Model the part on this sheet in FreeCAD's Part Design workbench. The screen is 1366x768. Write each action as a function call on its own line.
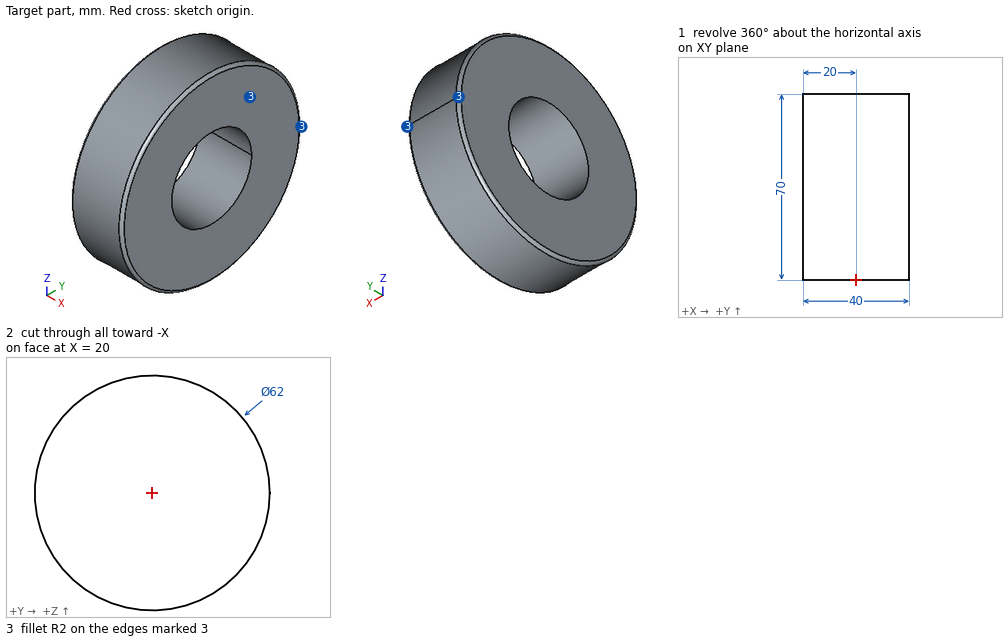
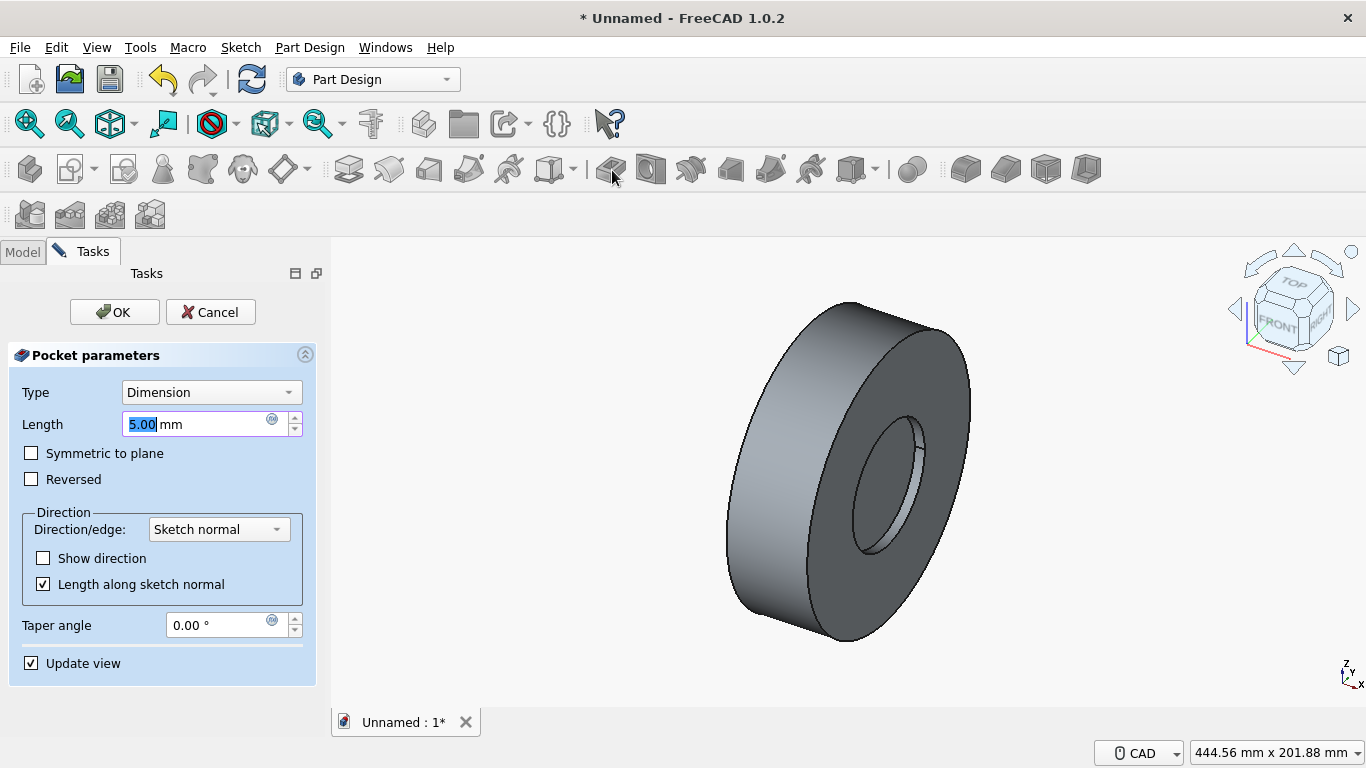
click(212, 392)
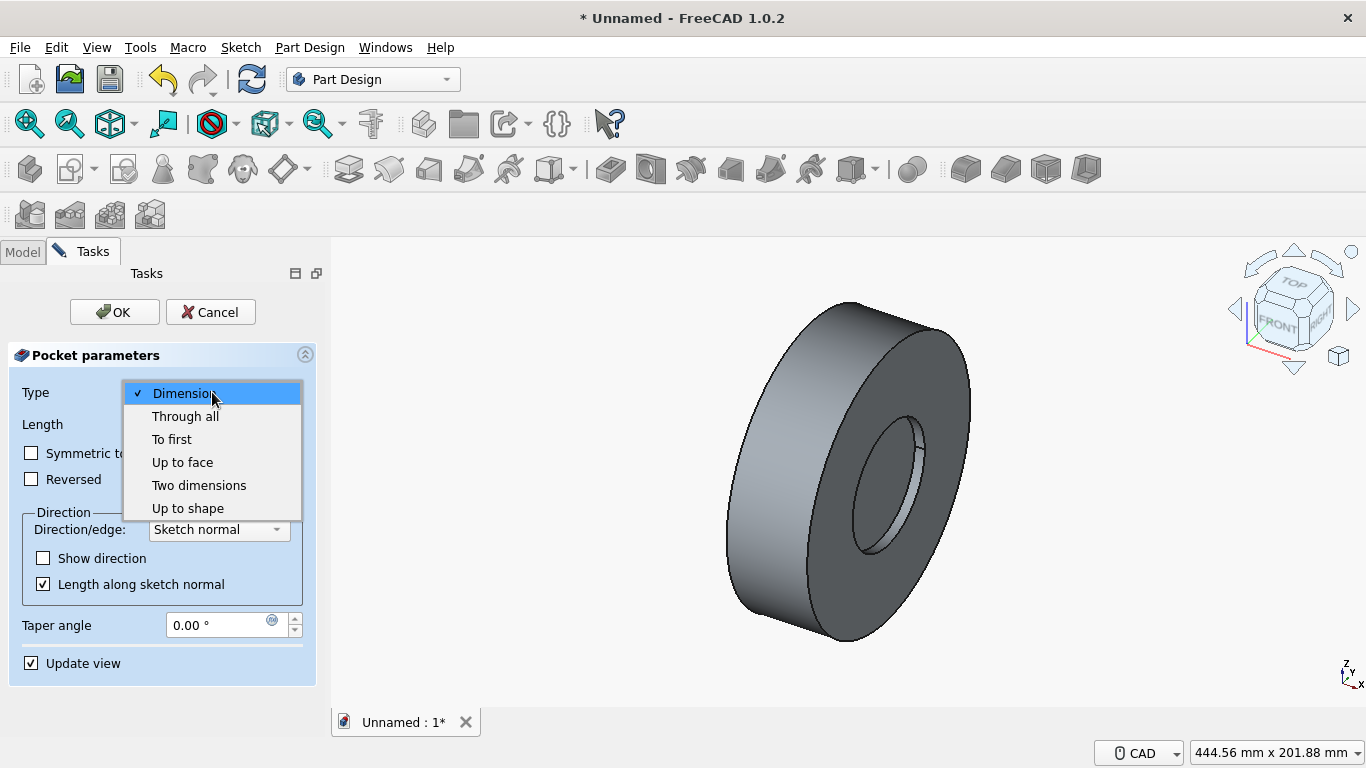
click(212, 416)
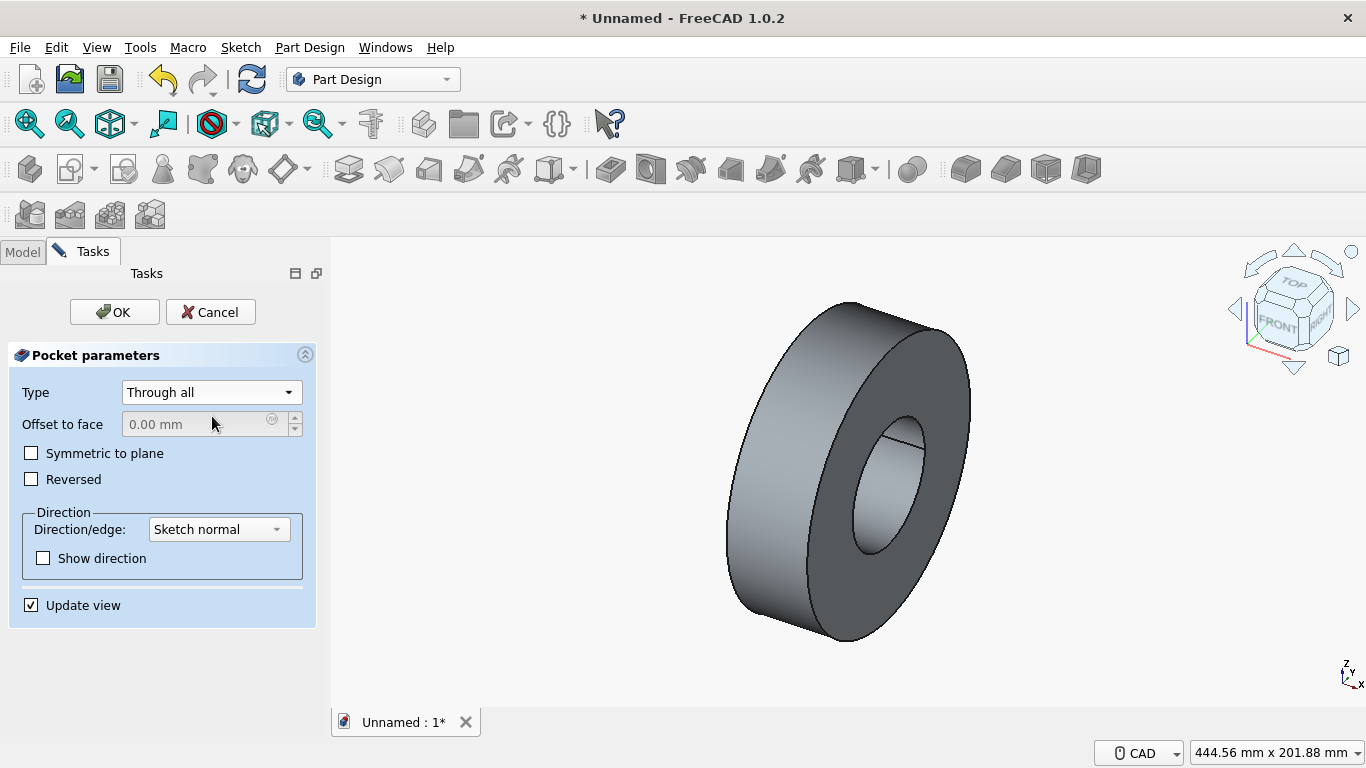
click(115, 312)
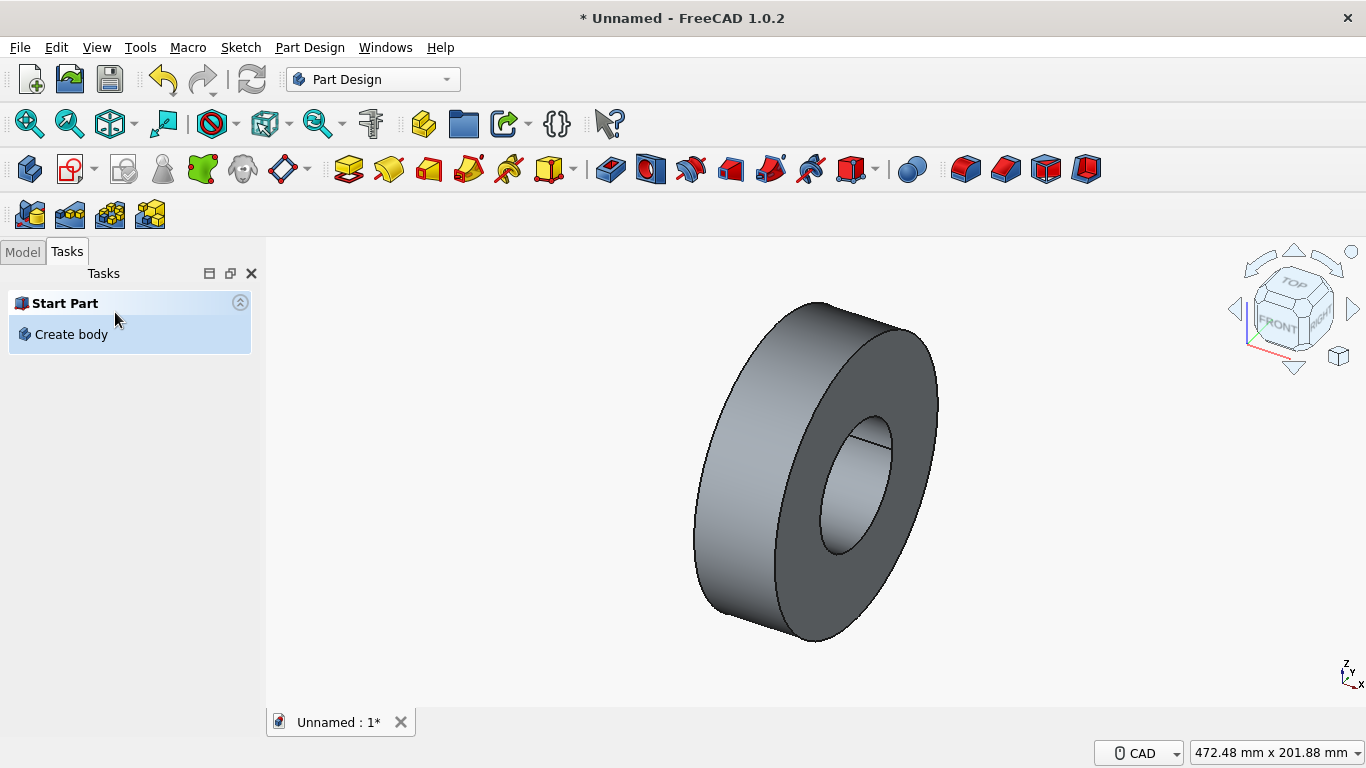
click(775, 565)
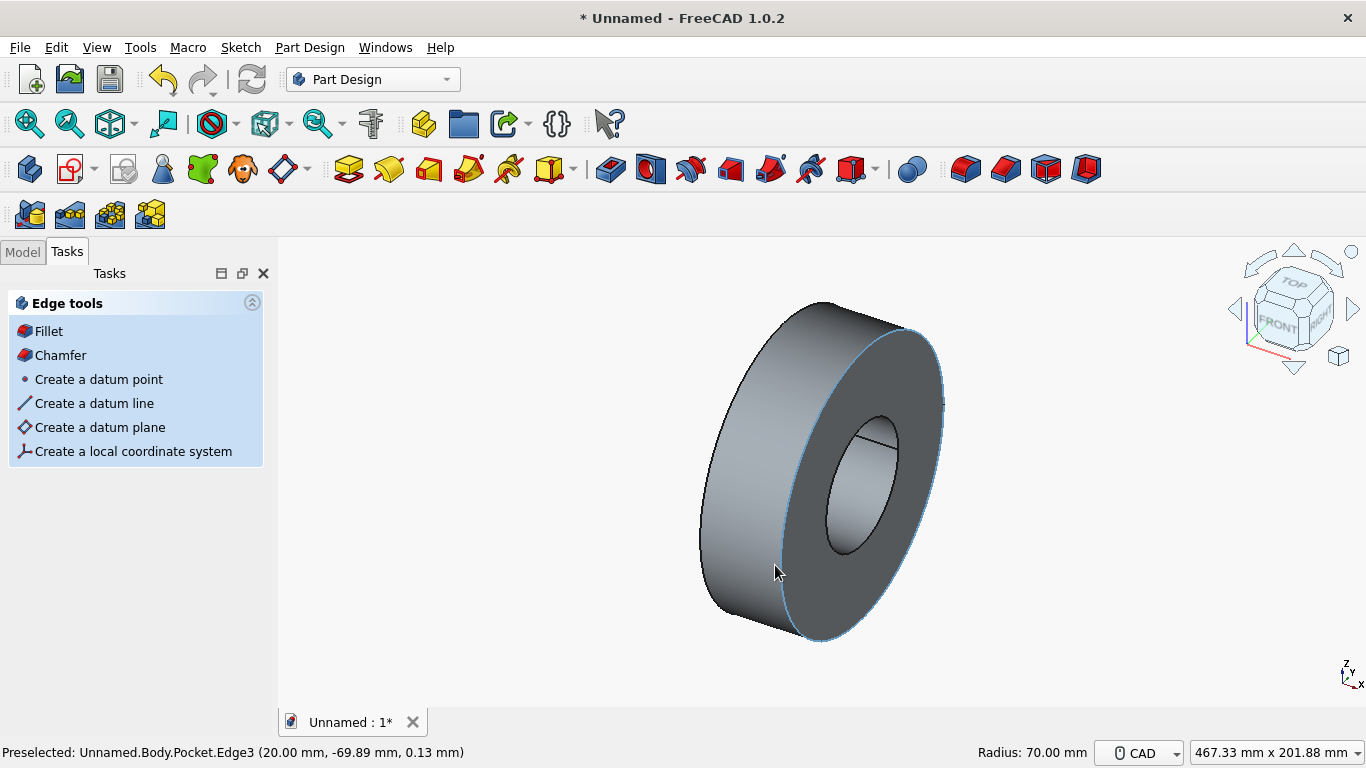
key(0)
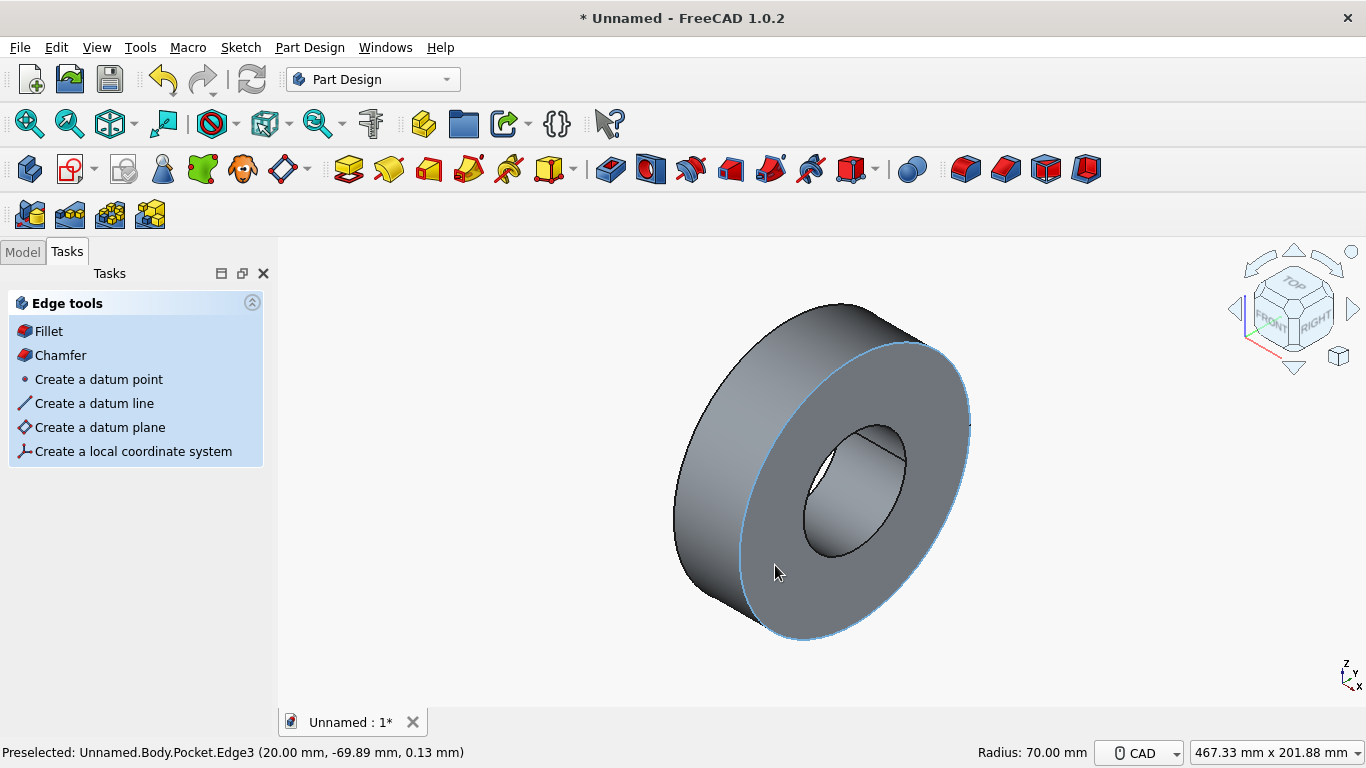
key(2)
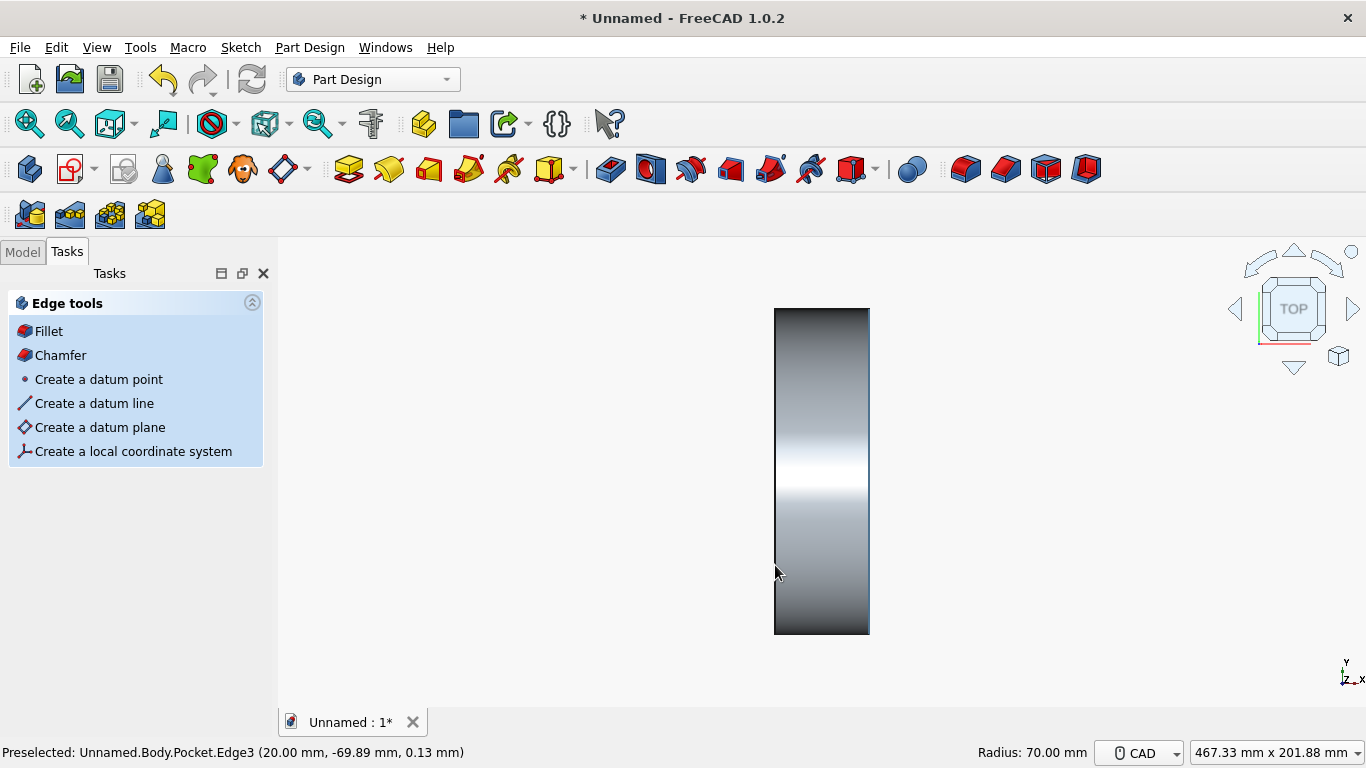
click(775, 603, ctrl)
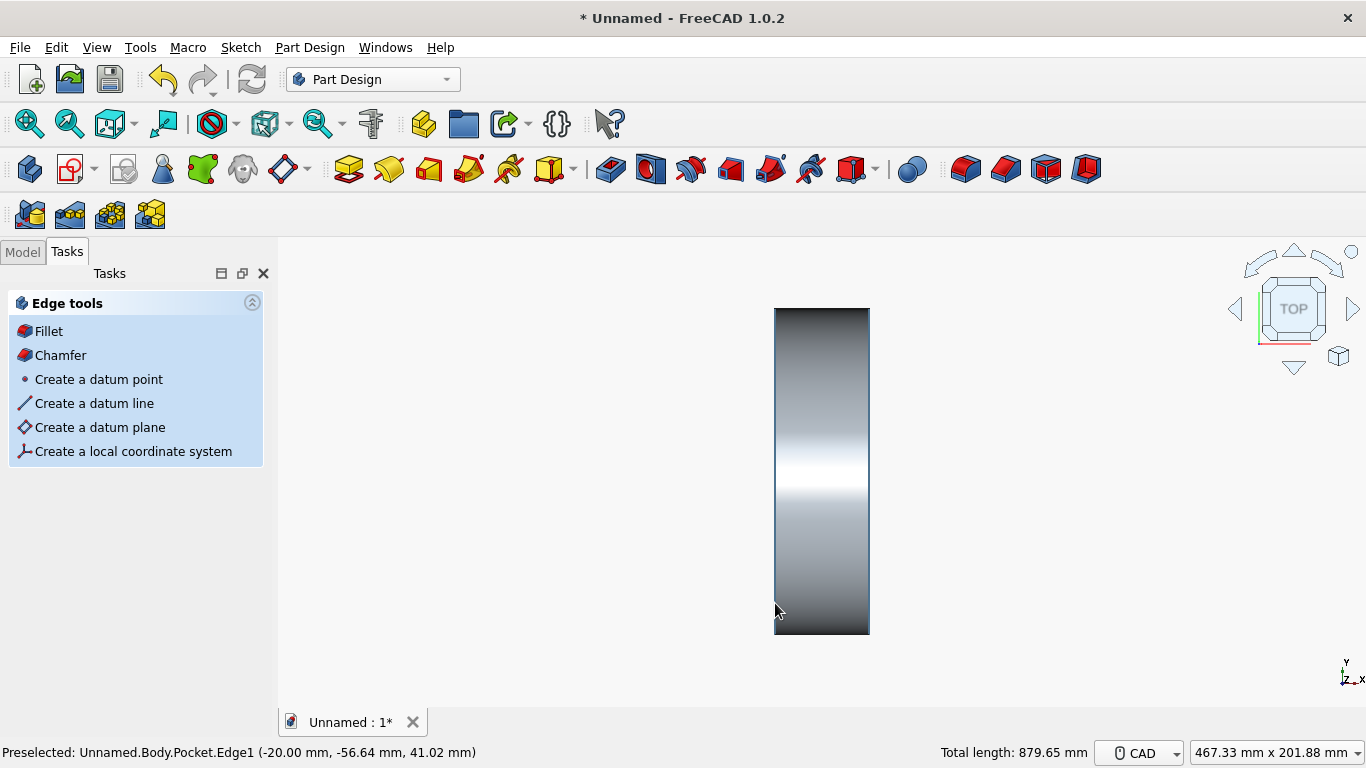
click(966, 170)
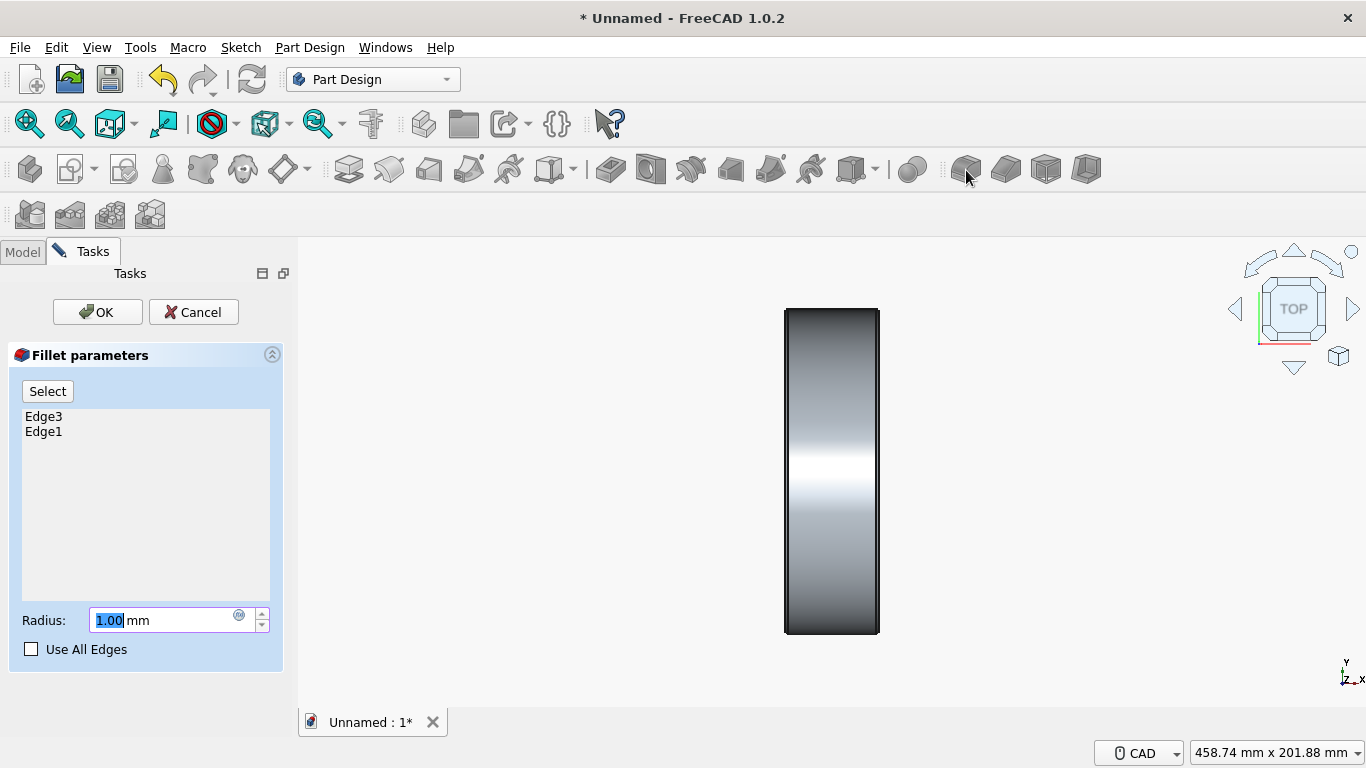
text(2)
key(Tab)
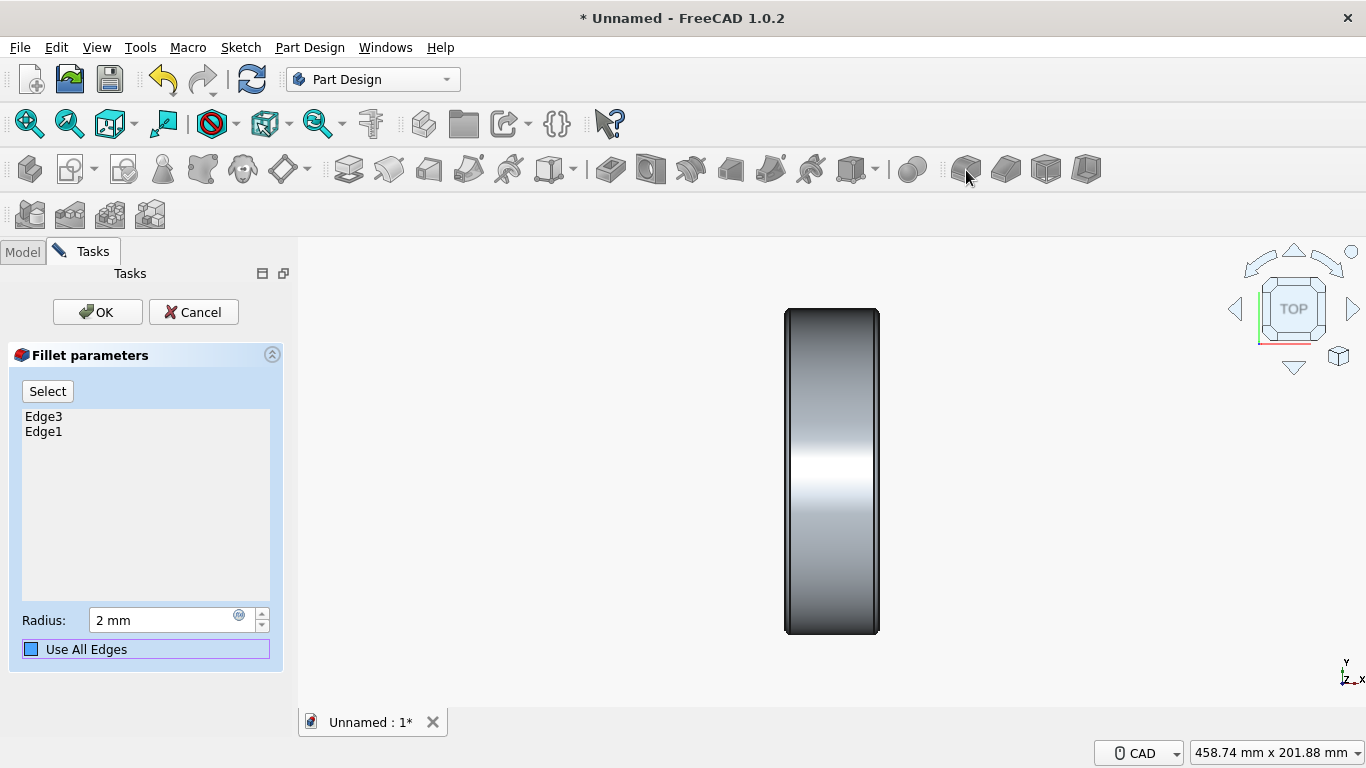
click(98, 312)